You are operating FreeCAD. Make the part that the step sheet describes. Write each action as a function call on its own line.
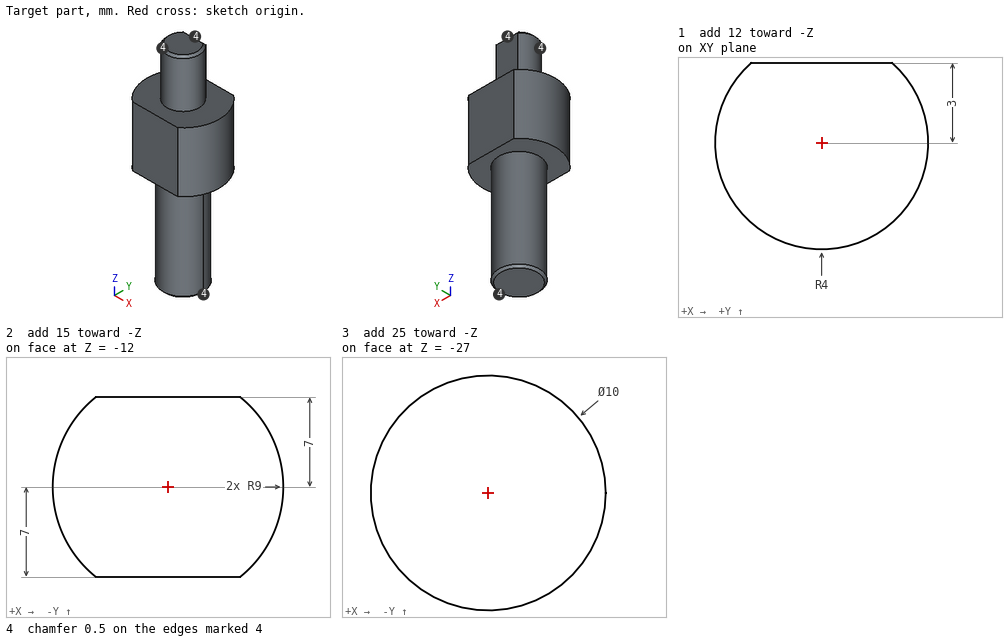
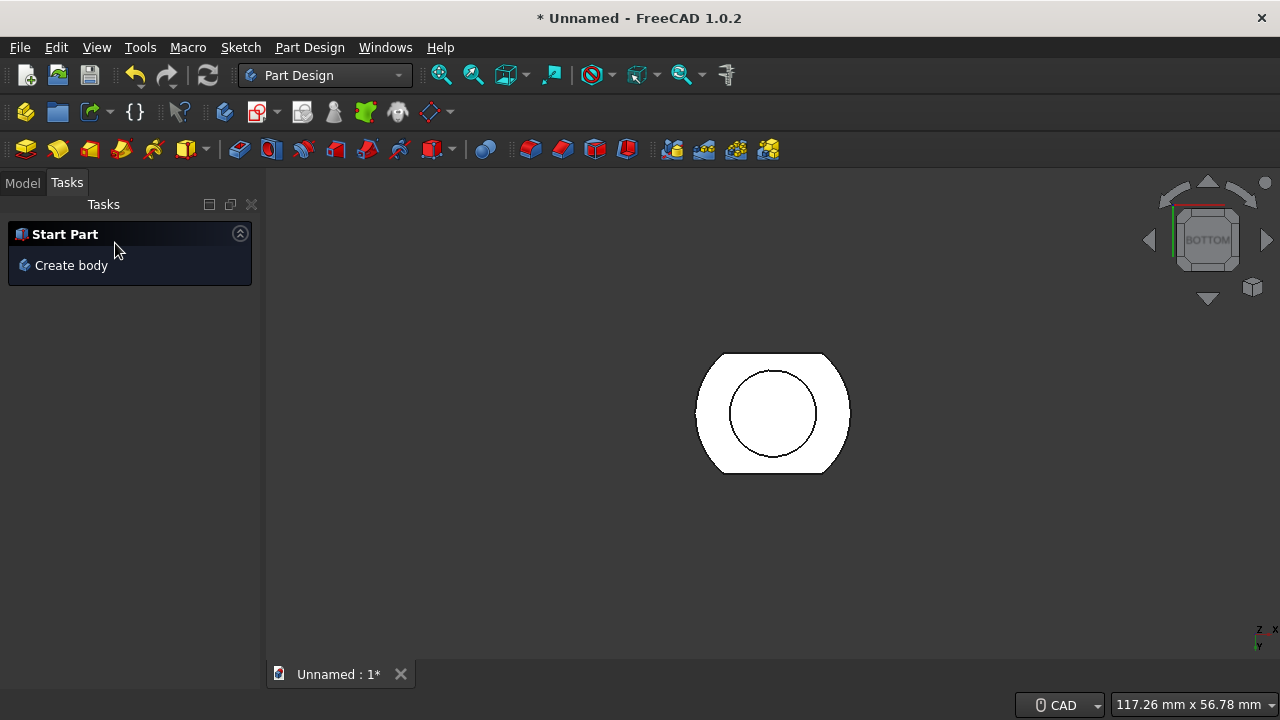
click(730, 412)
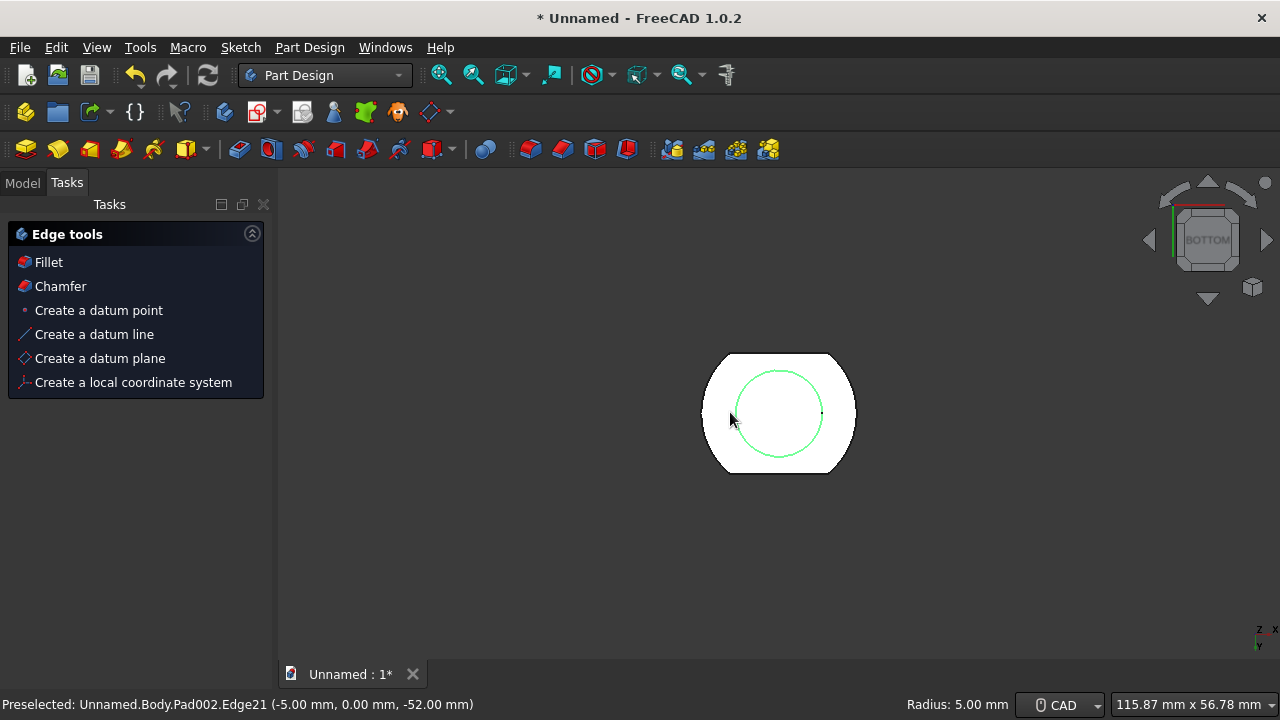
key(0)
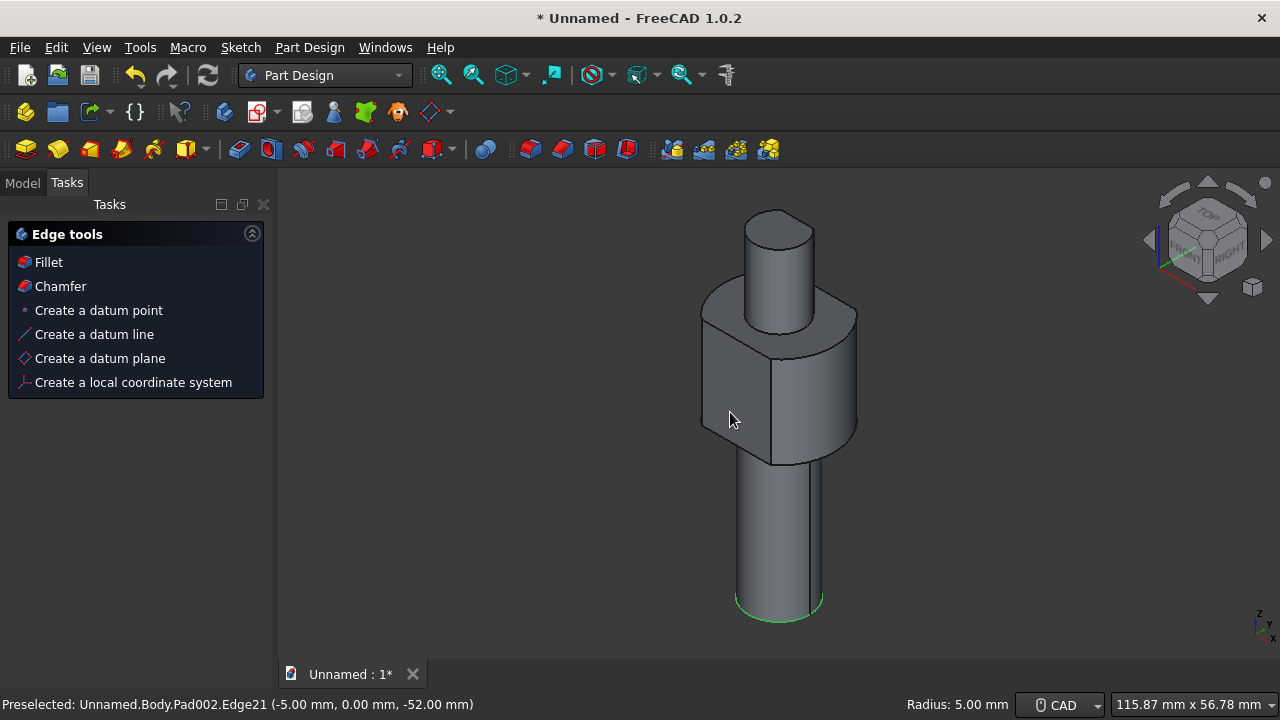
click(755, 243, ctrl)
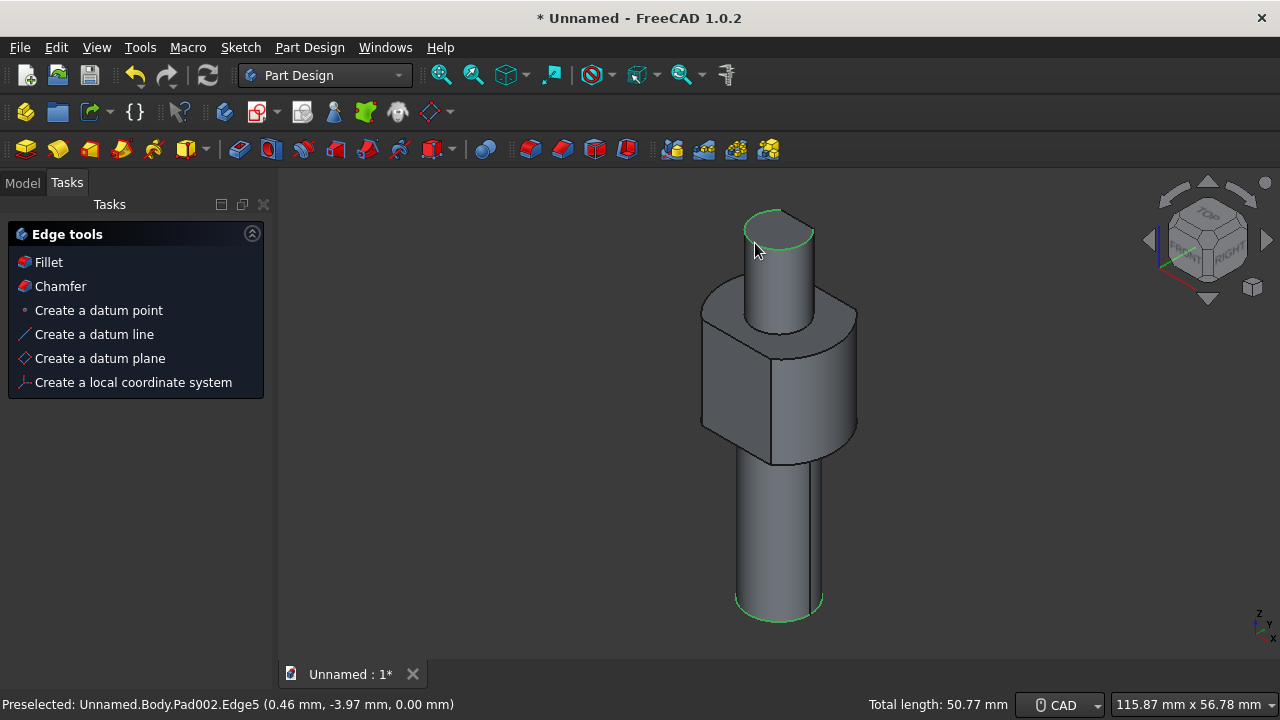
key(2)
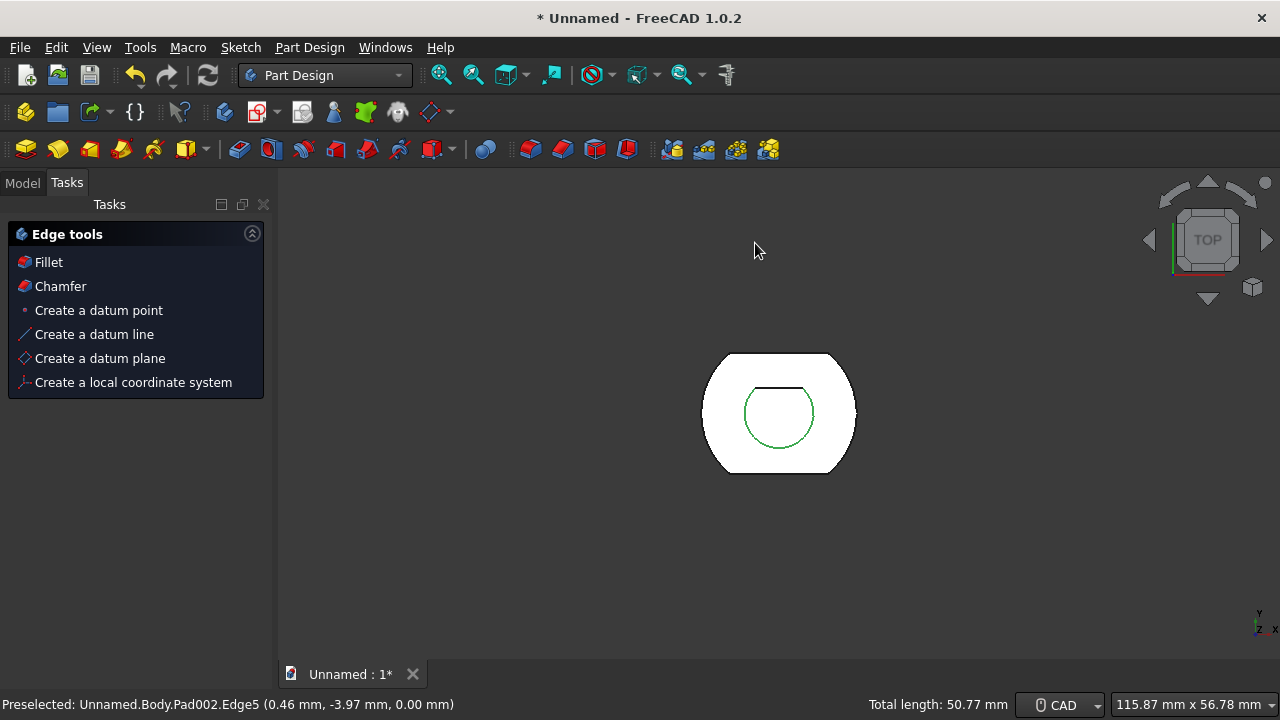
key(v)
key(f)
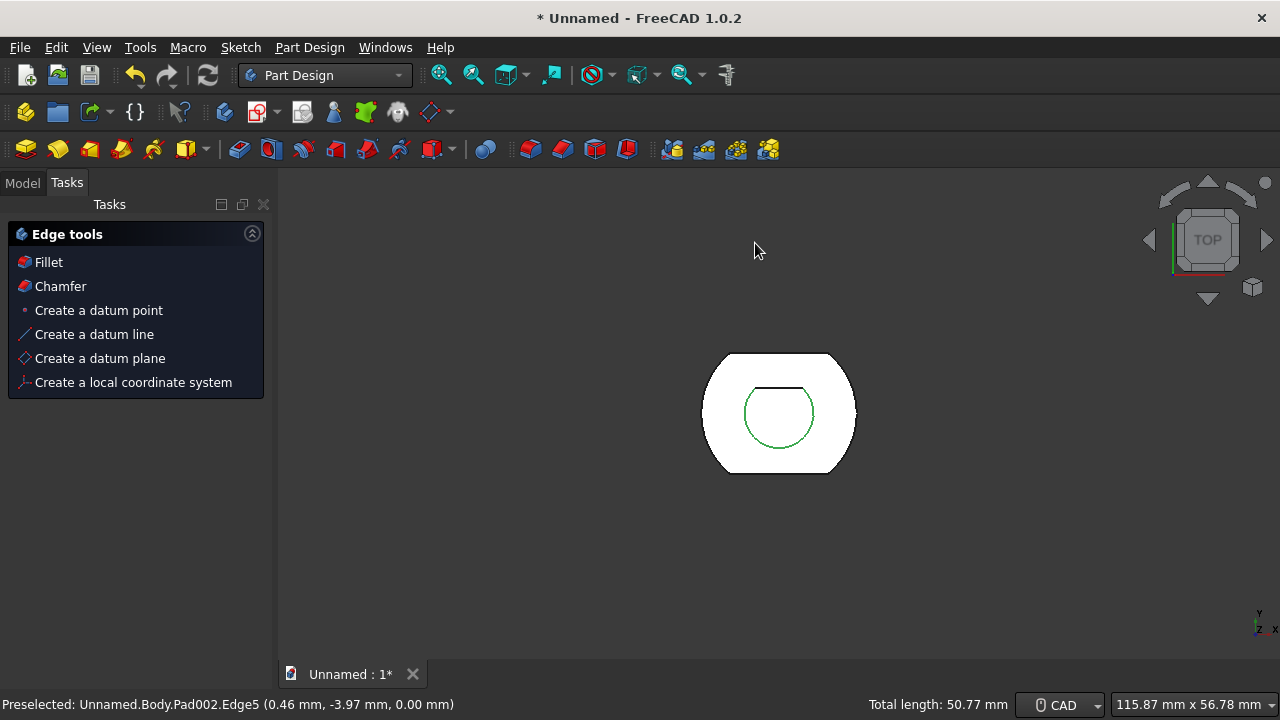
click(779, 387, ctrl)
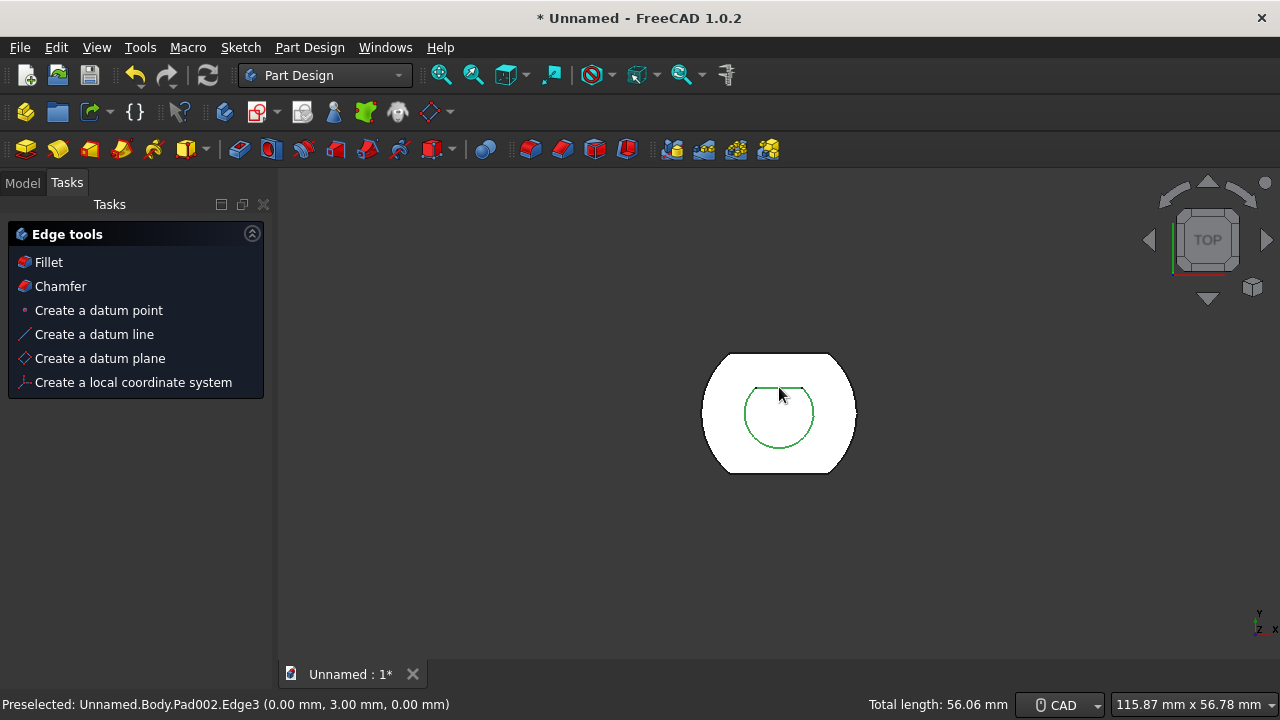
click(564, 150)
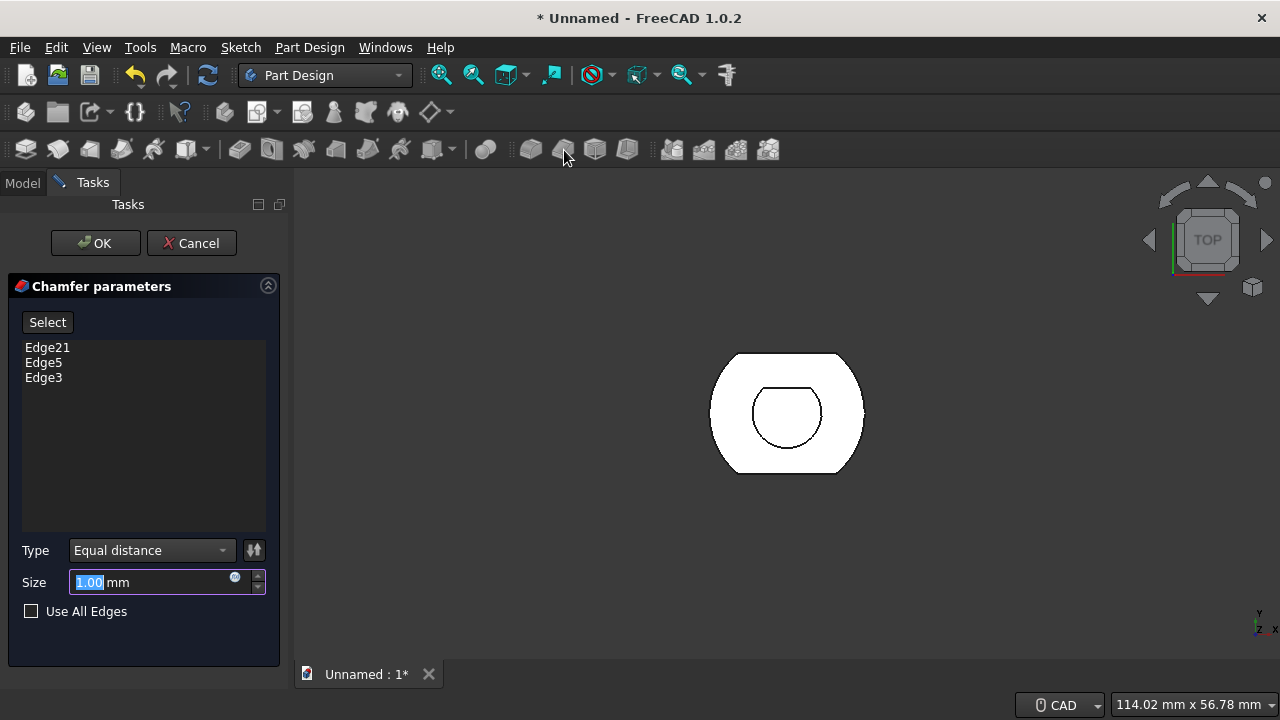
text(0.5)
key(Tab)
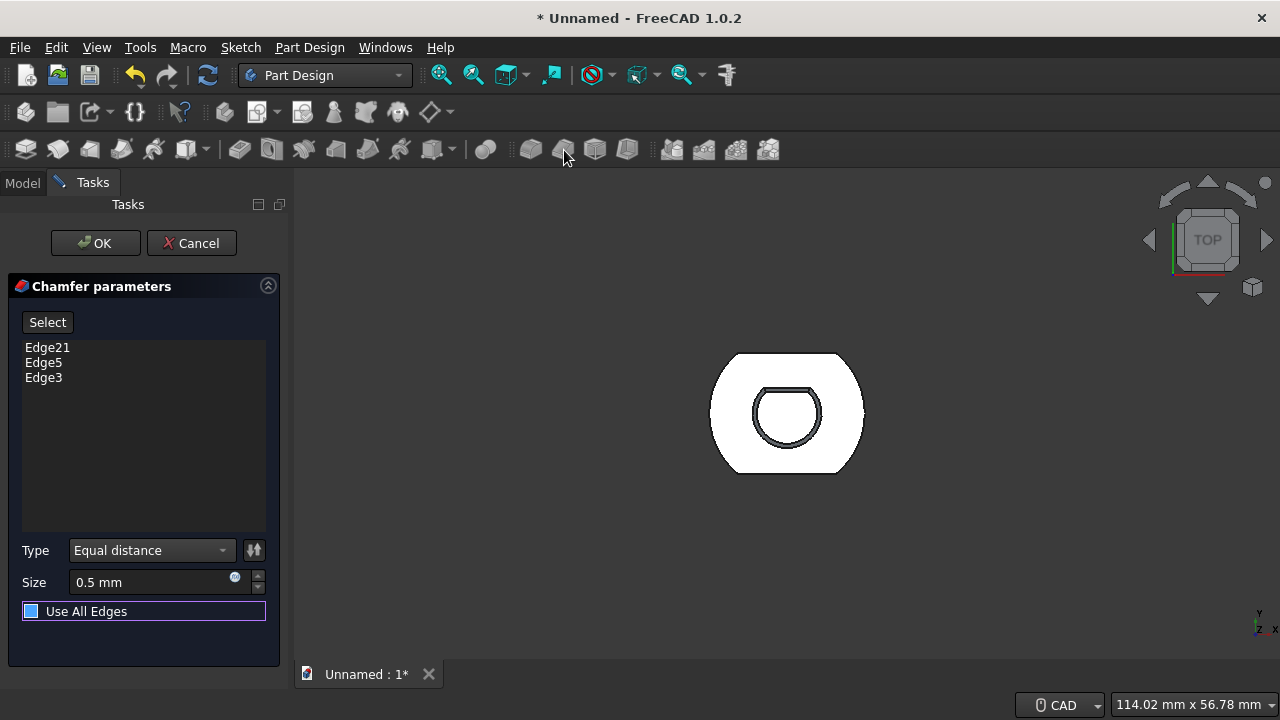
click(96, 243)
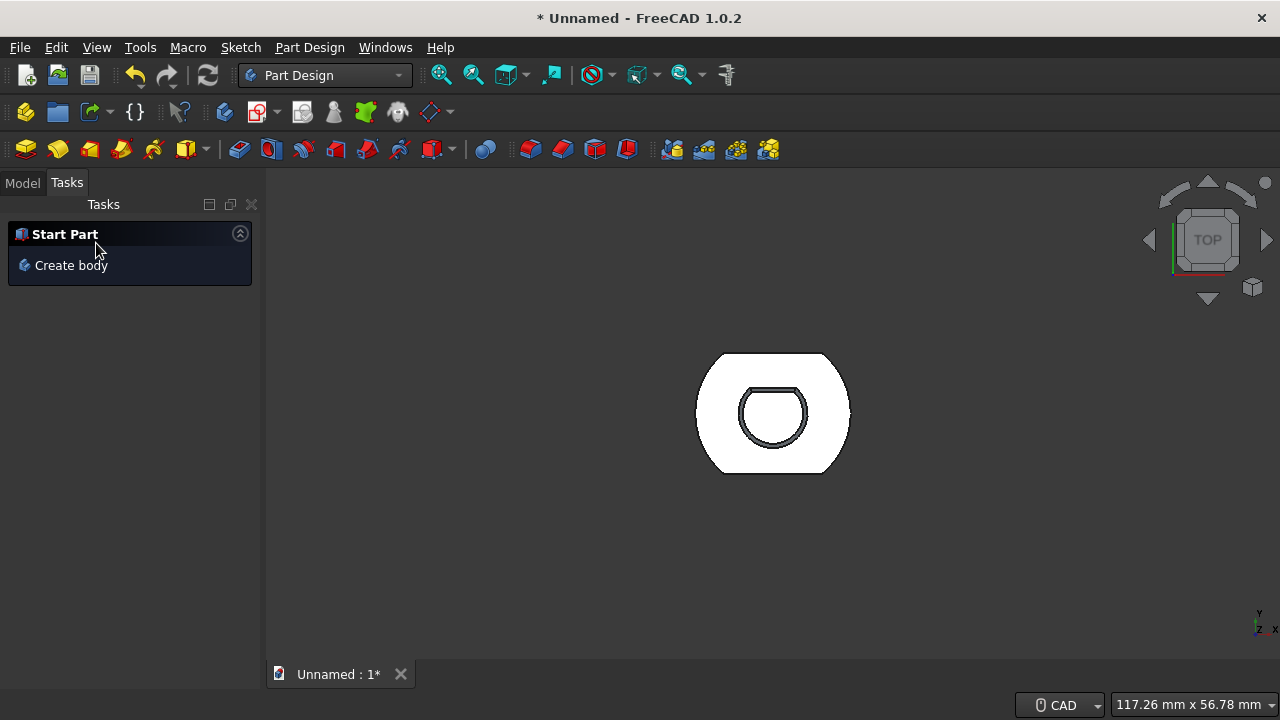
key(0)